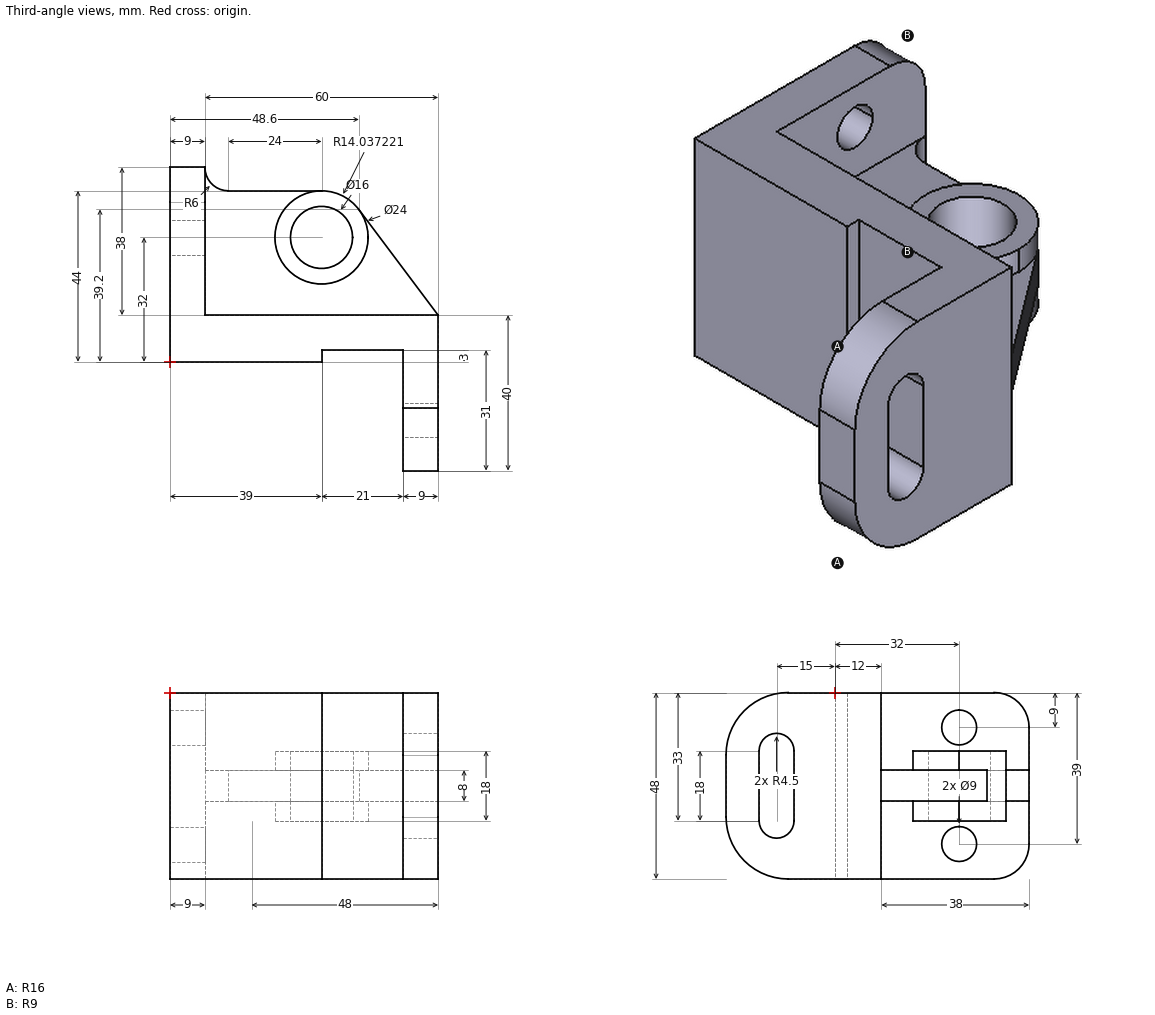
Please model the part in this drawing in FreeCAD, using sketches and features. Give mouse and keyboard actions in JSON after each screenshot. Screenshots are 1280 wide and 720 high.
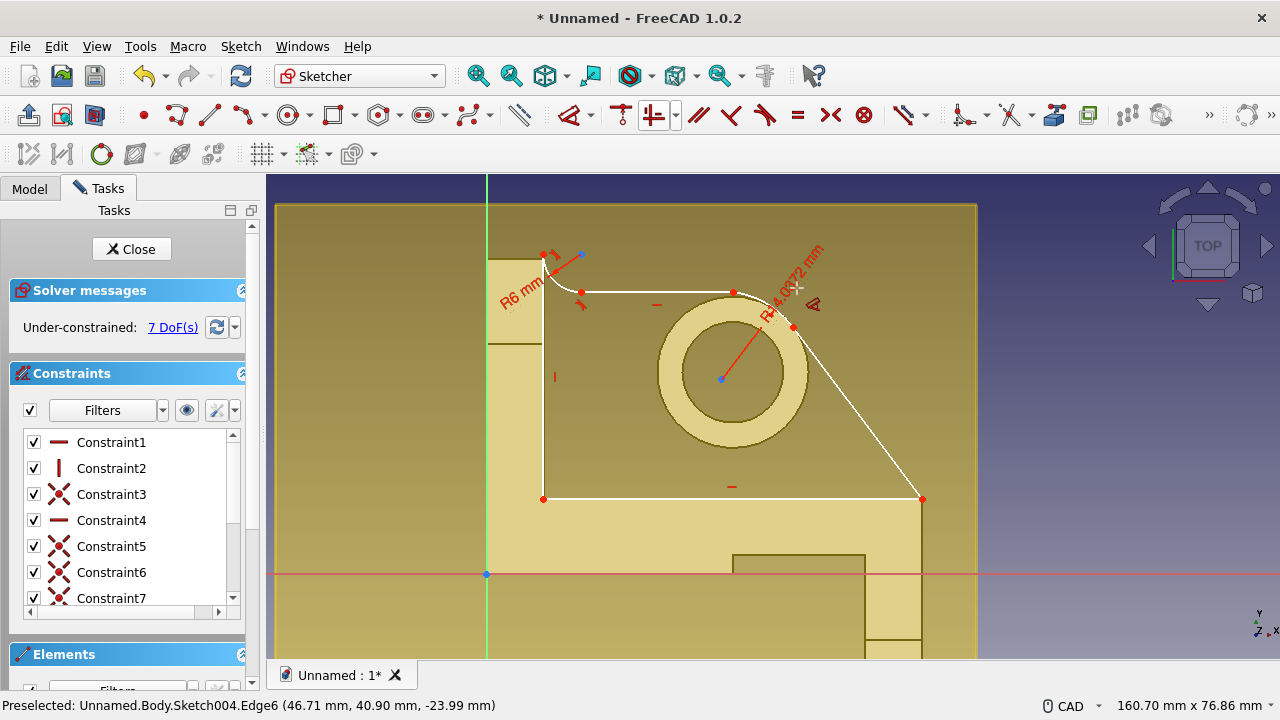
{"action": "left_click", "coordinate": [688, 292]}
{"action": "left_click", "coordinate": [657, 258]}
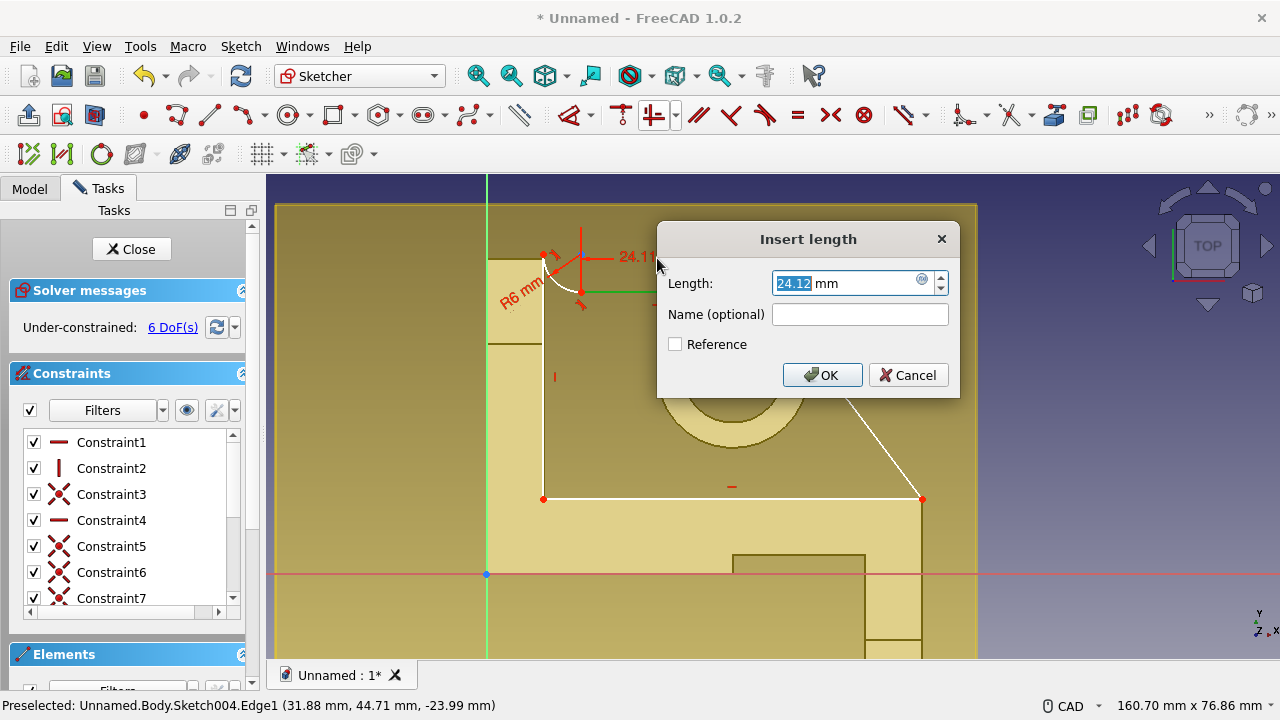
{"action": "type", "text": "24"}
{"action": "key", "text": "Return"}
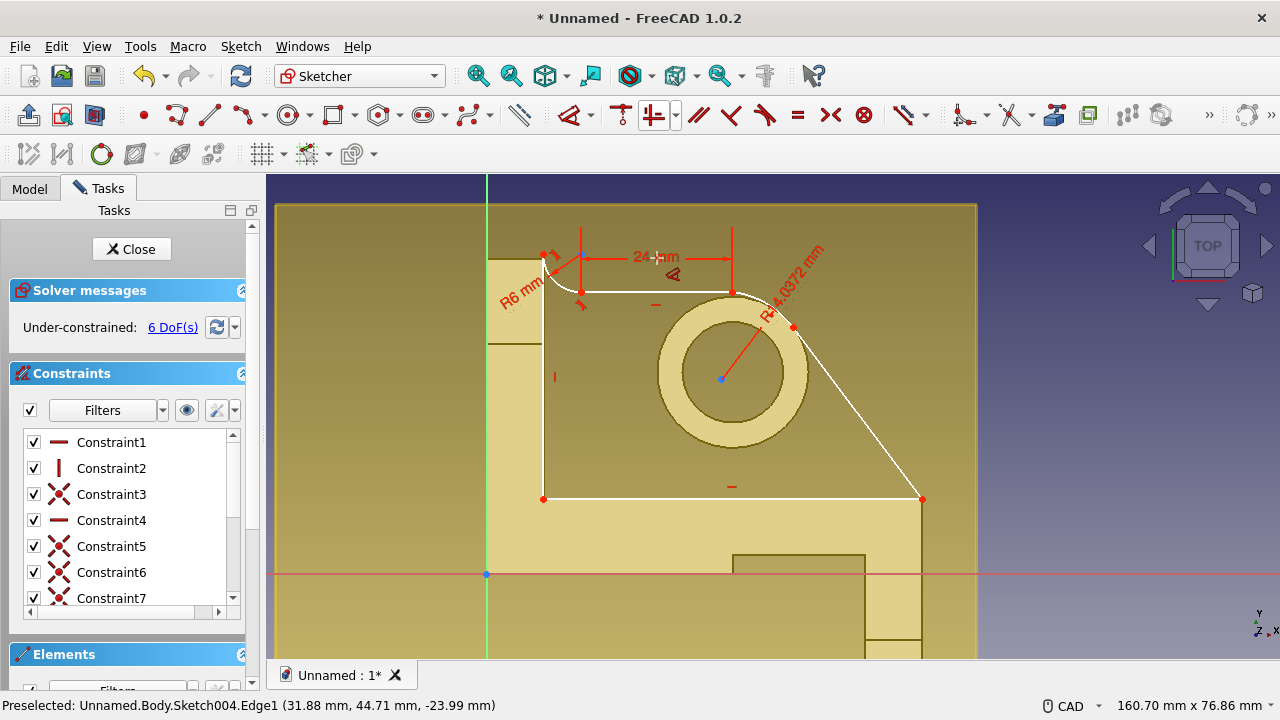
{"action": "left_click", "coordinate": [543, 328]}
{"action": "left_click", "coordinate": [509, 377]}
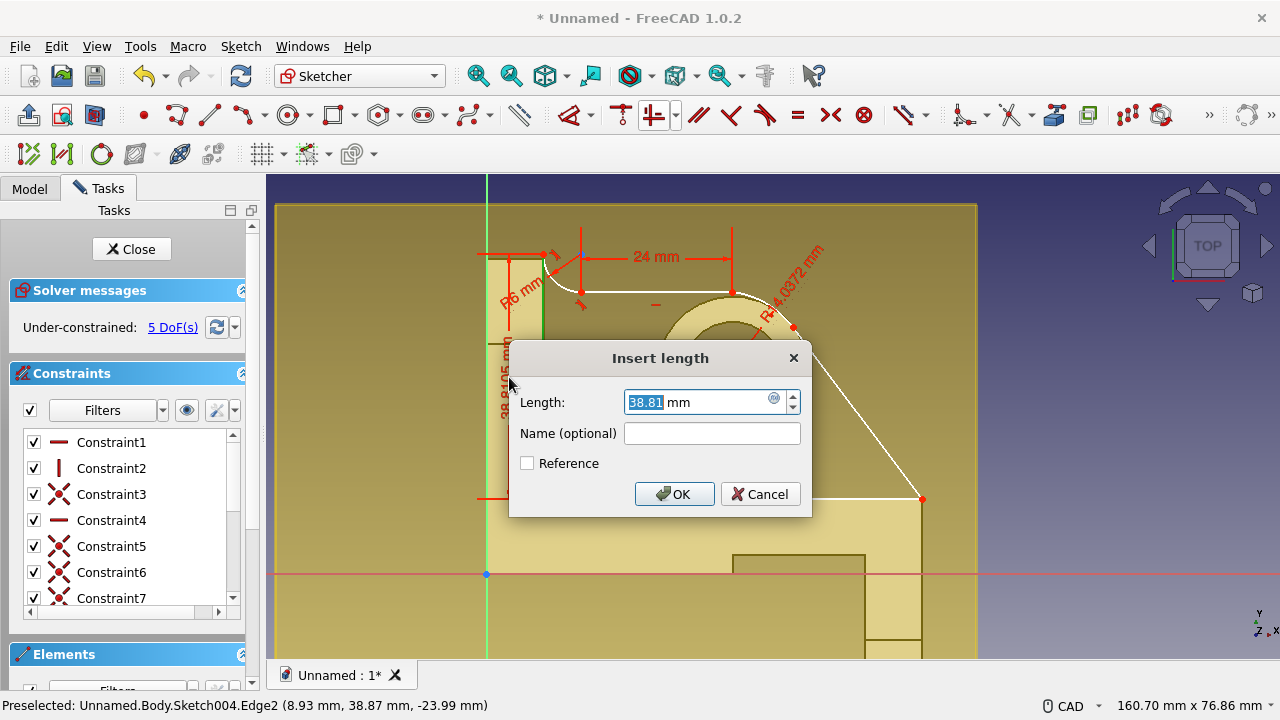
{"action": "type", "text": "38"}
{"action": "key", "text": "Return"}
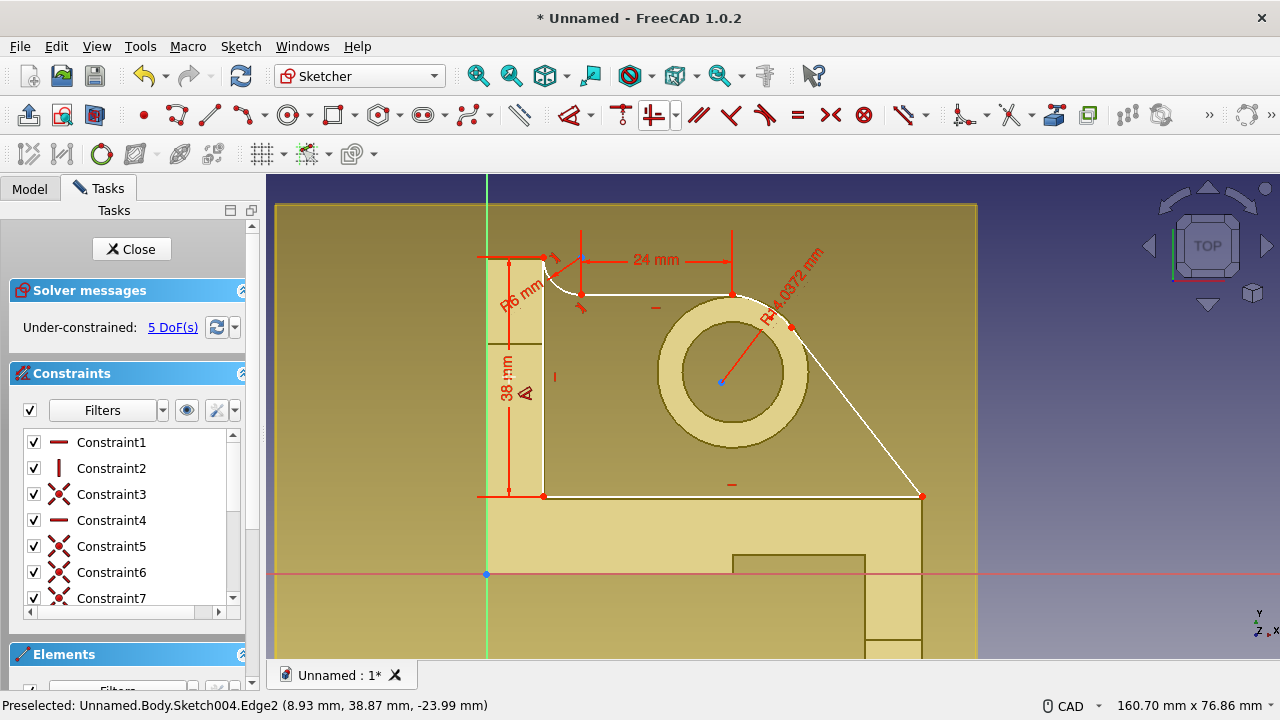
{"action": "left_click", "coordinate": [657, 497]}
{"action": "left_click", "coordinate": [733, 531]}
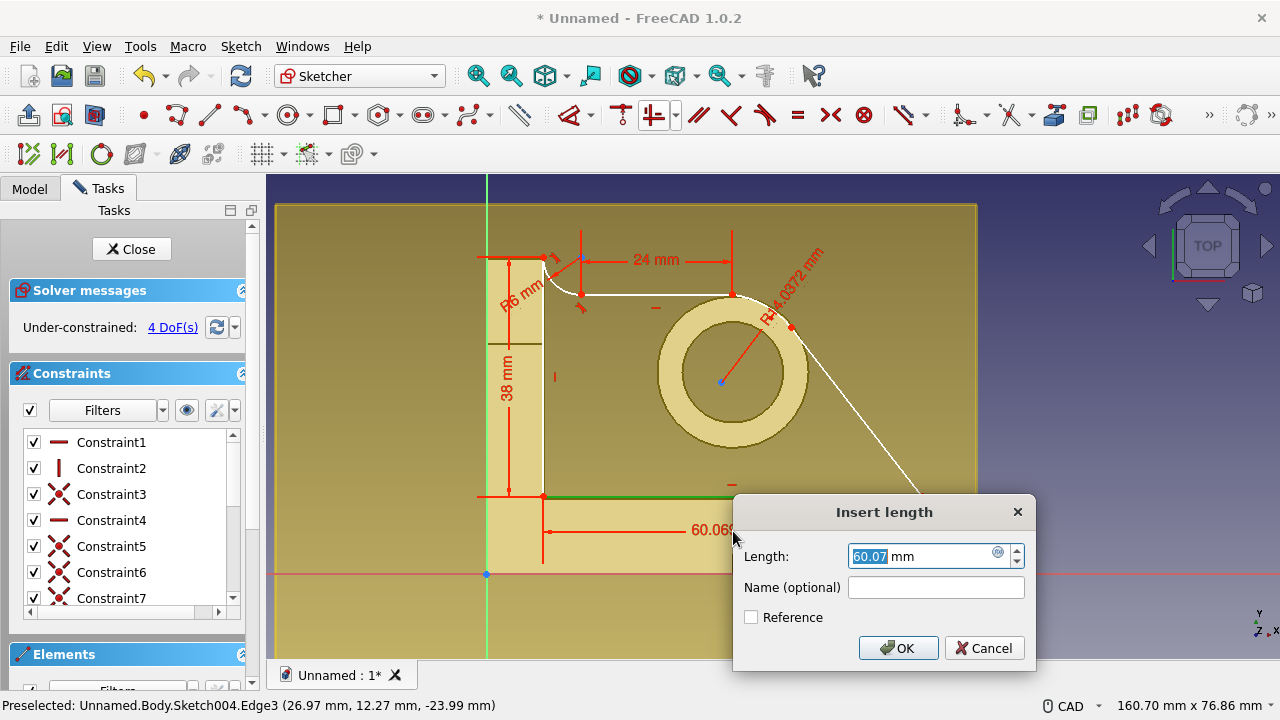
{"action": "type", "text": "60"}
{"action": "key", "text": "Return"}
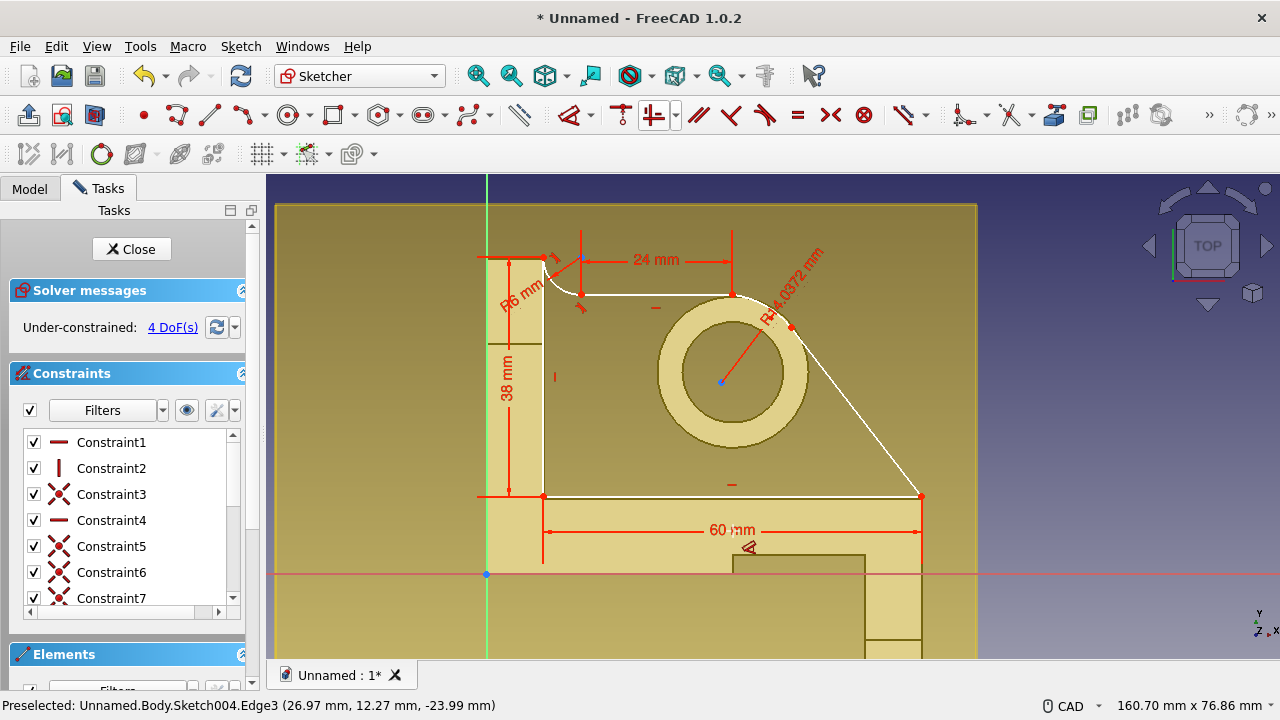
{"action": "left_click", "coordinate": [543, 257]}
{"action": "left_click", "coordinate": [515, 223]}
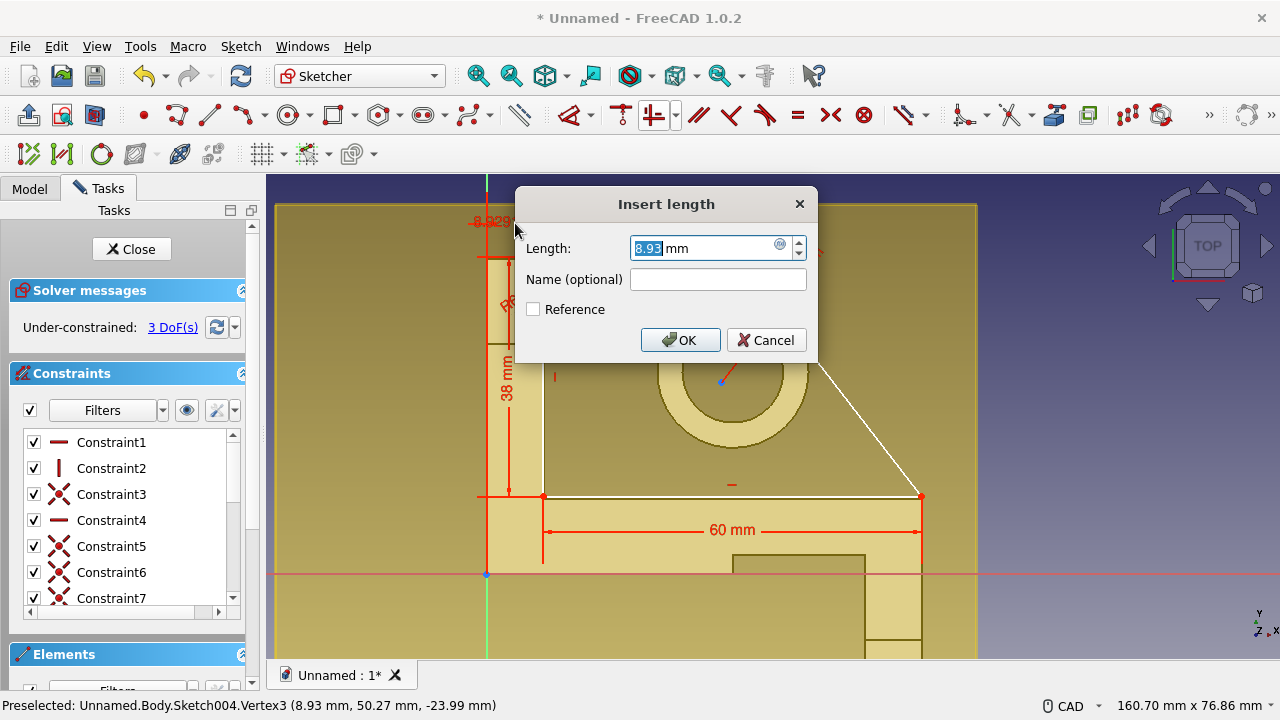
{"action": "type", "text": "9"}
{"action": "key", "text": "Return"}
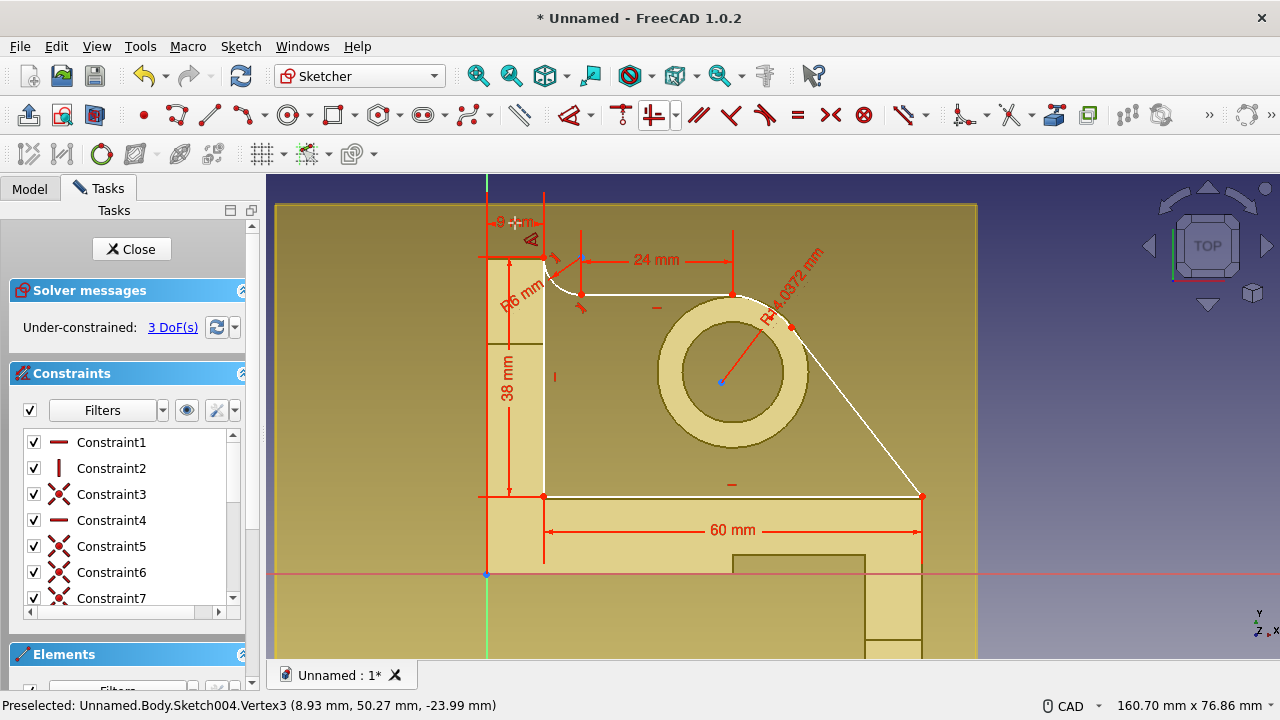
{"action": "left_click", "coordinate": [733, 295]}
{"action": "left_click", "coordinate": [453, 435]}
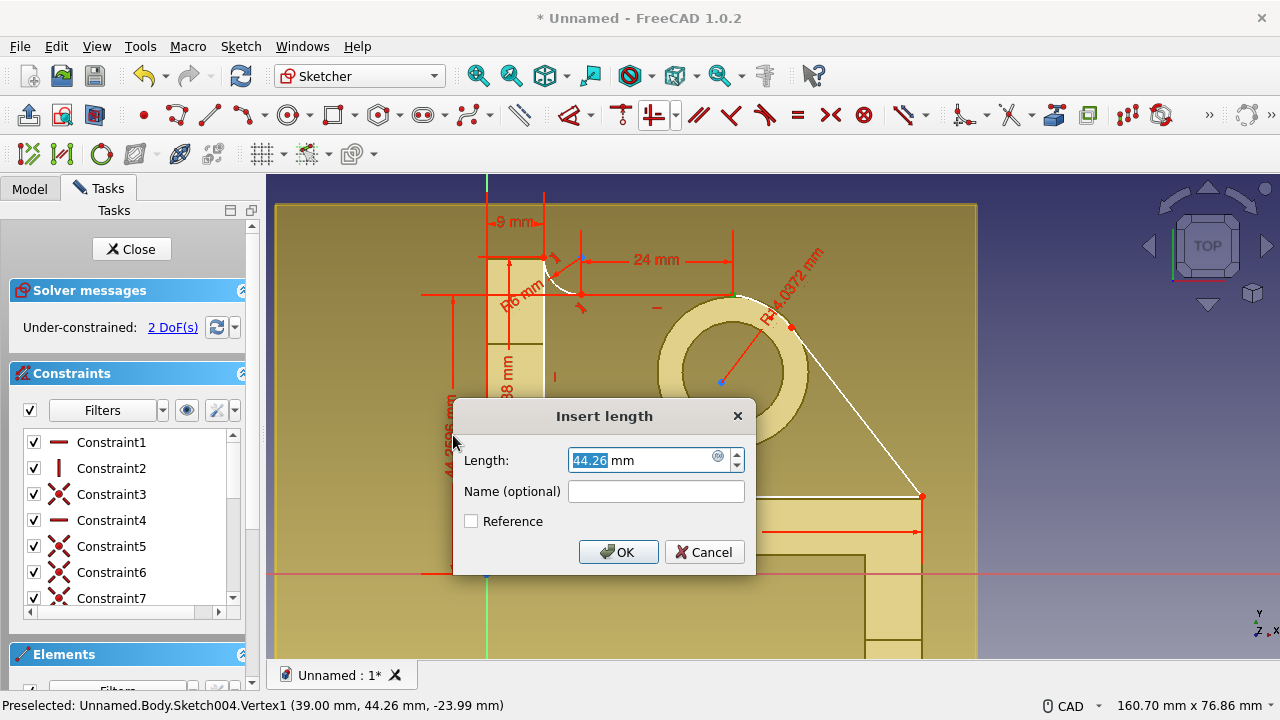
{"action": "type", "text": "44"}
{"action": "key", "text": "Return"}